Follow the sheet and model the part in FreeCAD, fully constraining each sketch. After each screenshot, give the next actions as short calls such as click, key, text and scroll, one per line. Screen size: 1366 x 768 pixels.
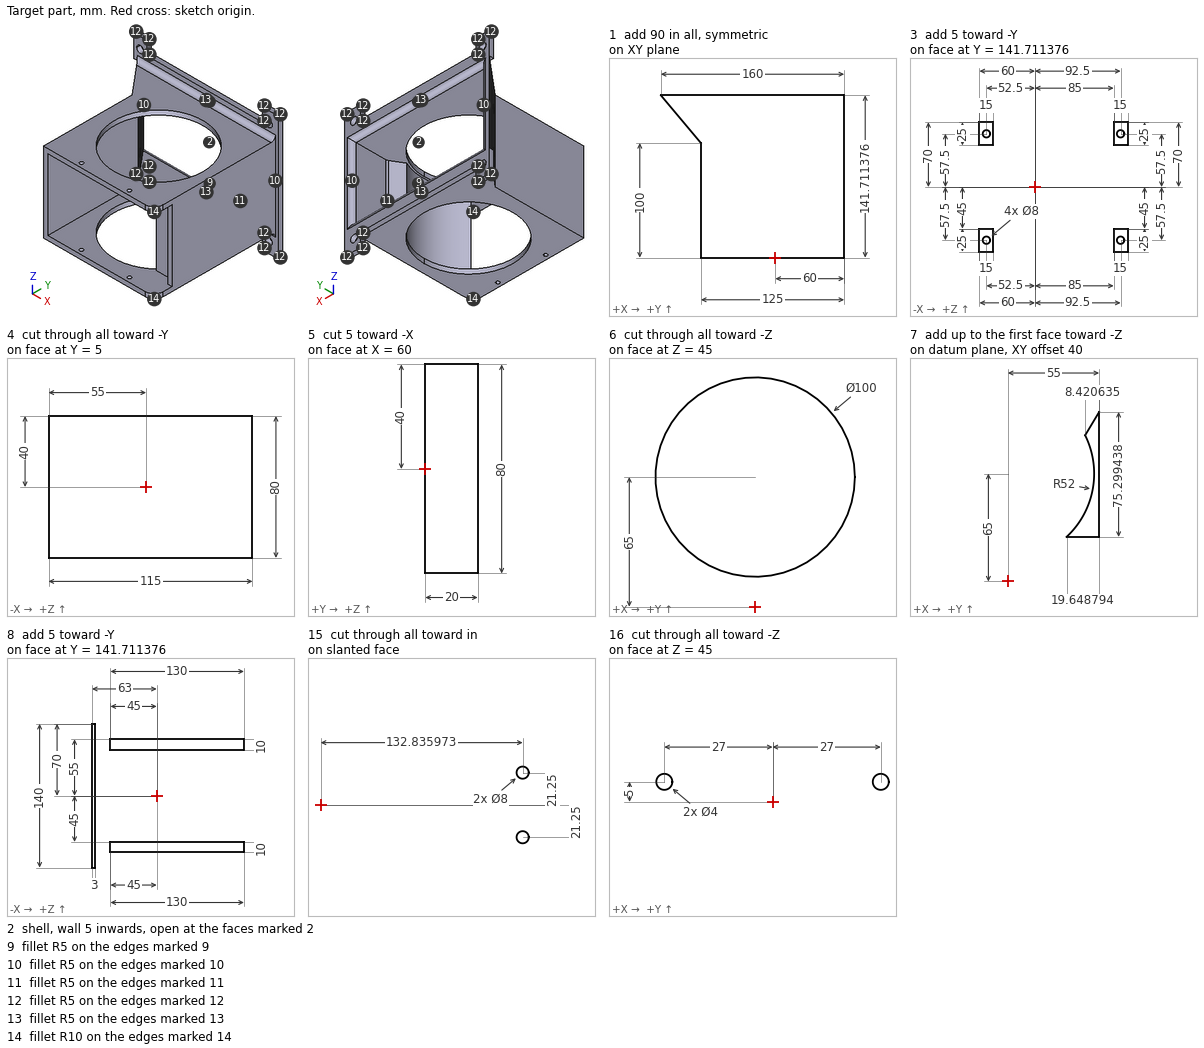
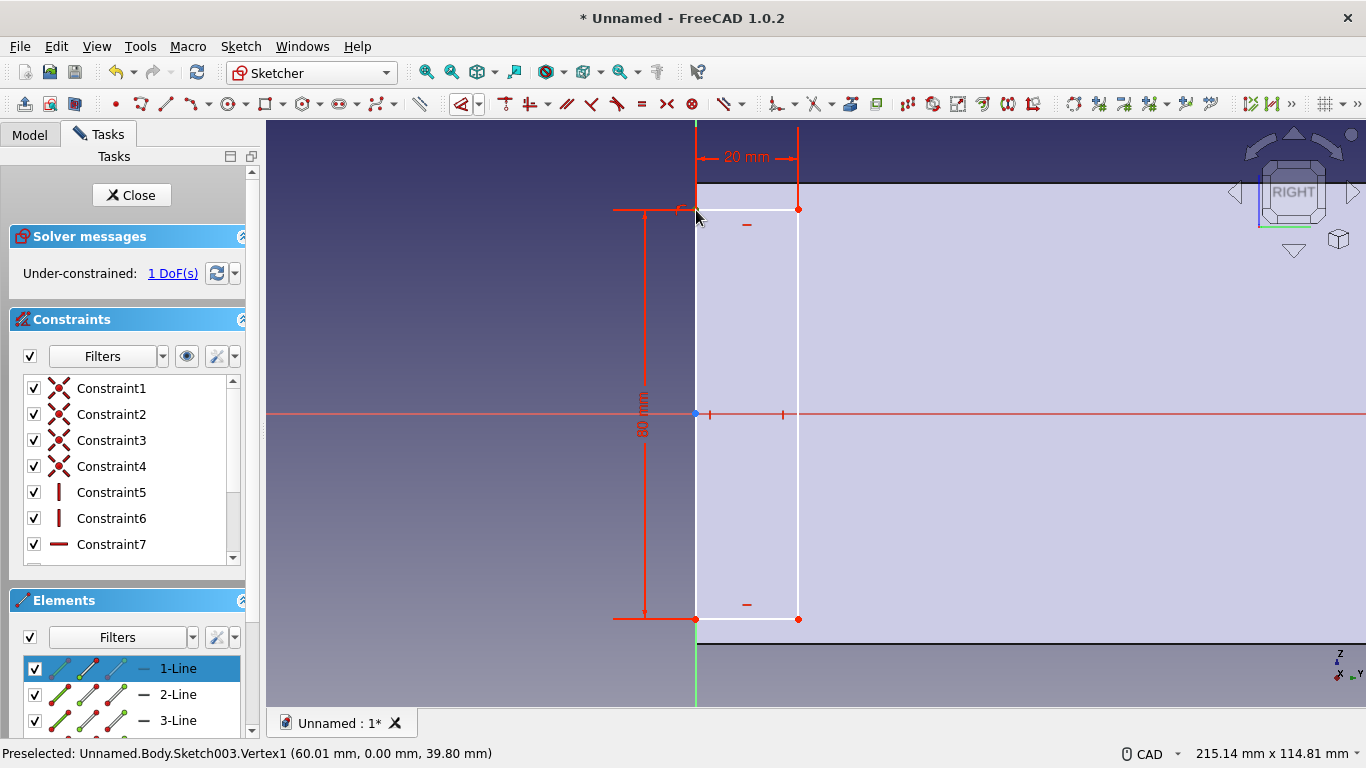
key(i)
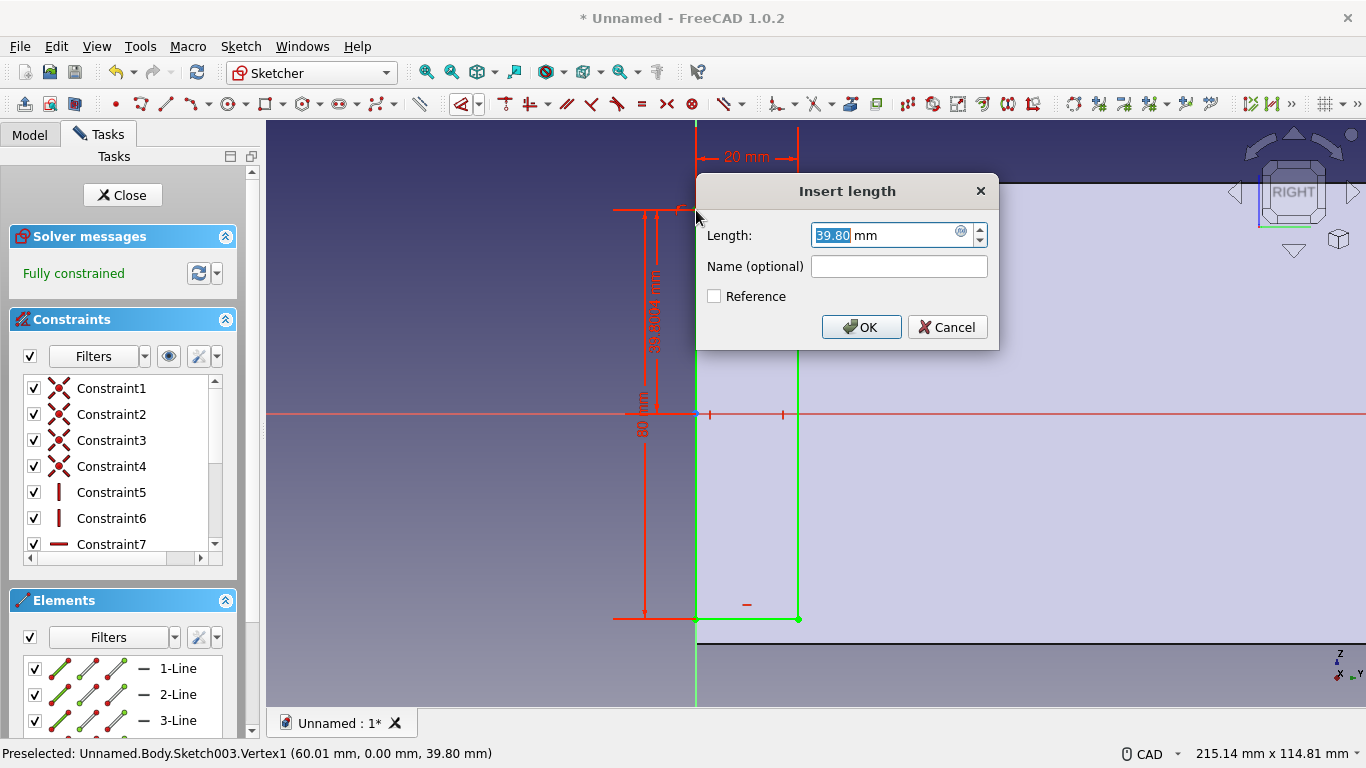
text(40)
key(Return)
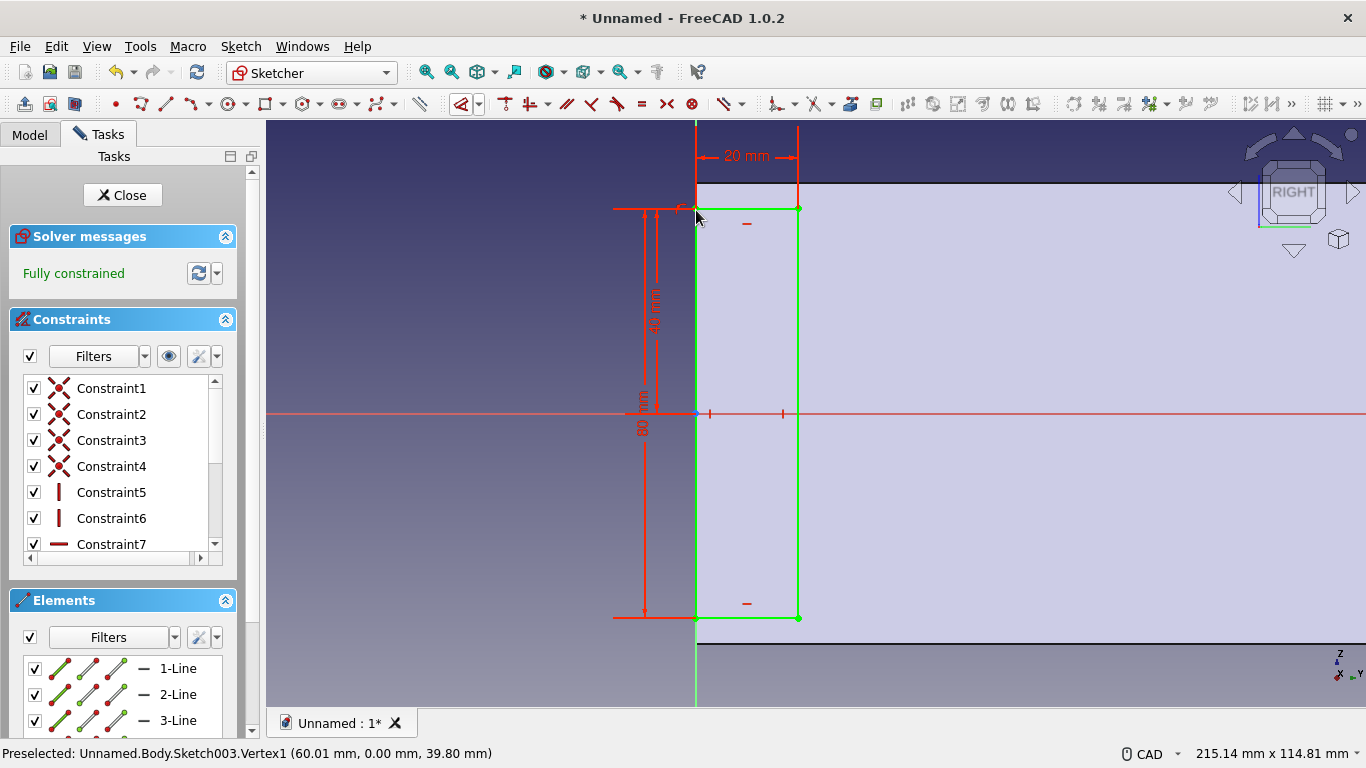
click(123, 195)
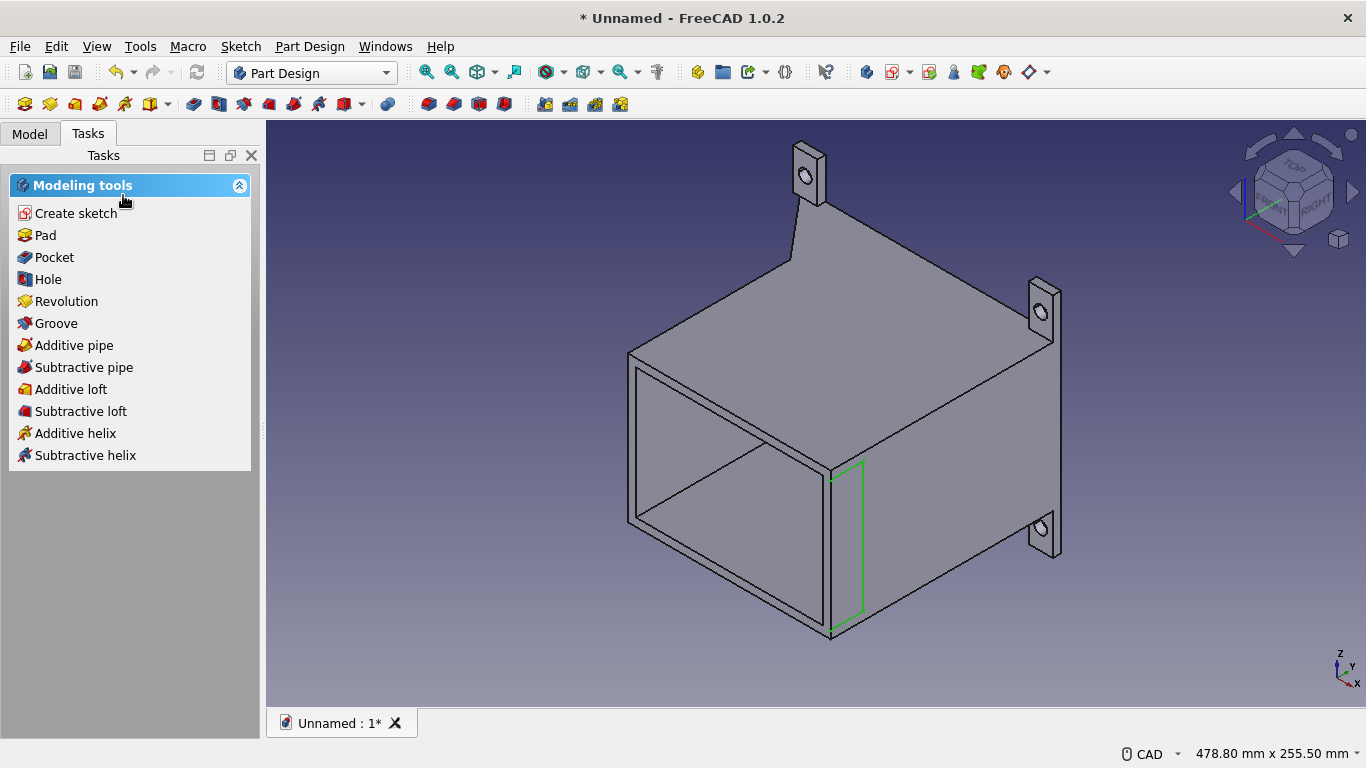
click(194, 104)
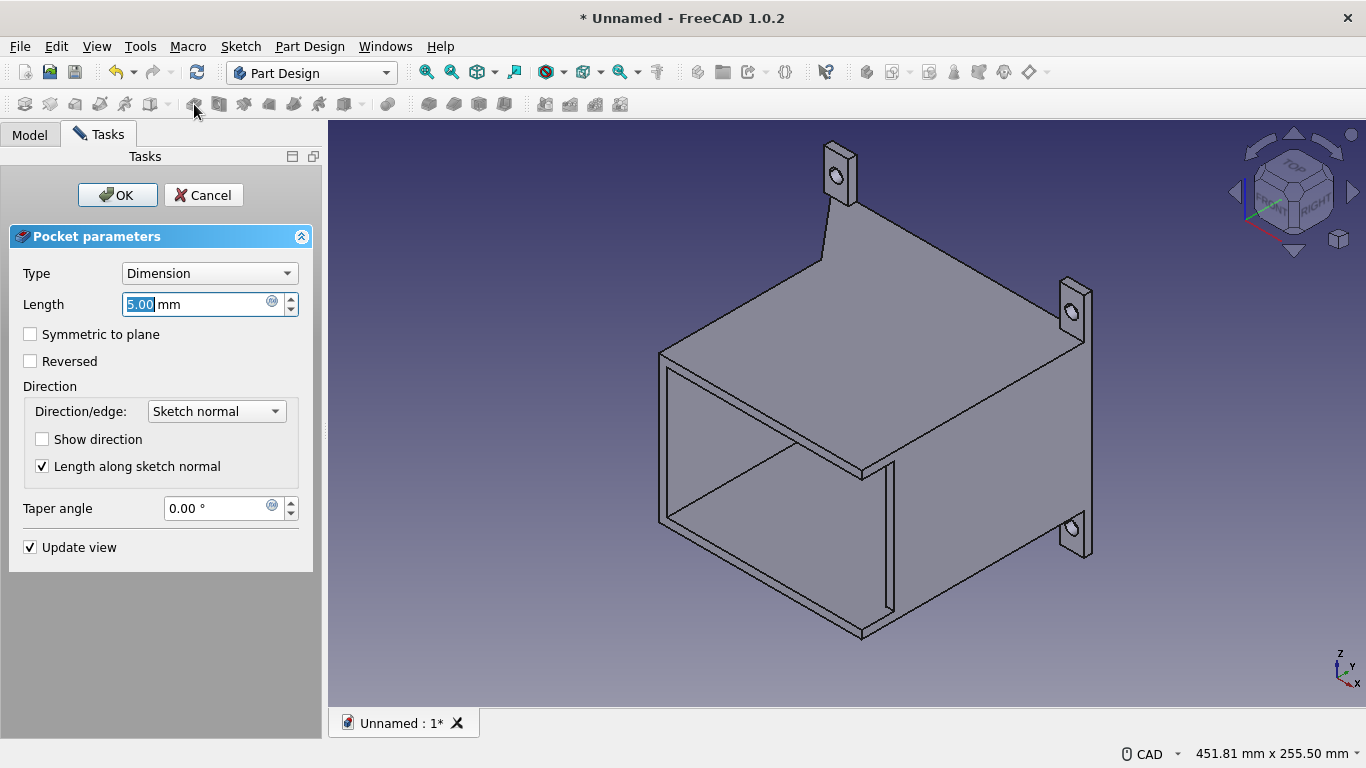
text(5)
key(Tab)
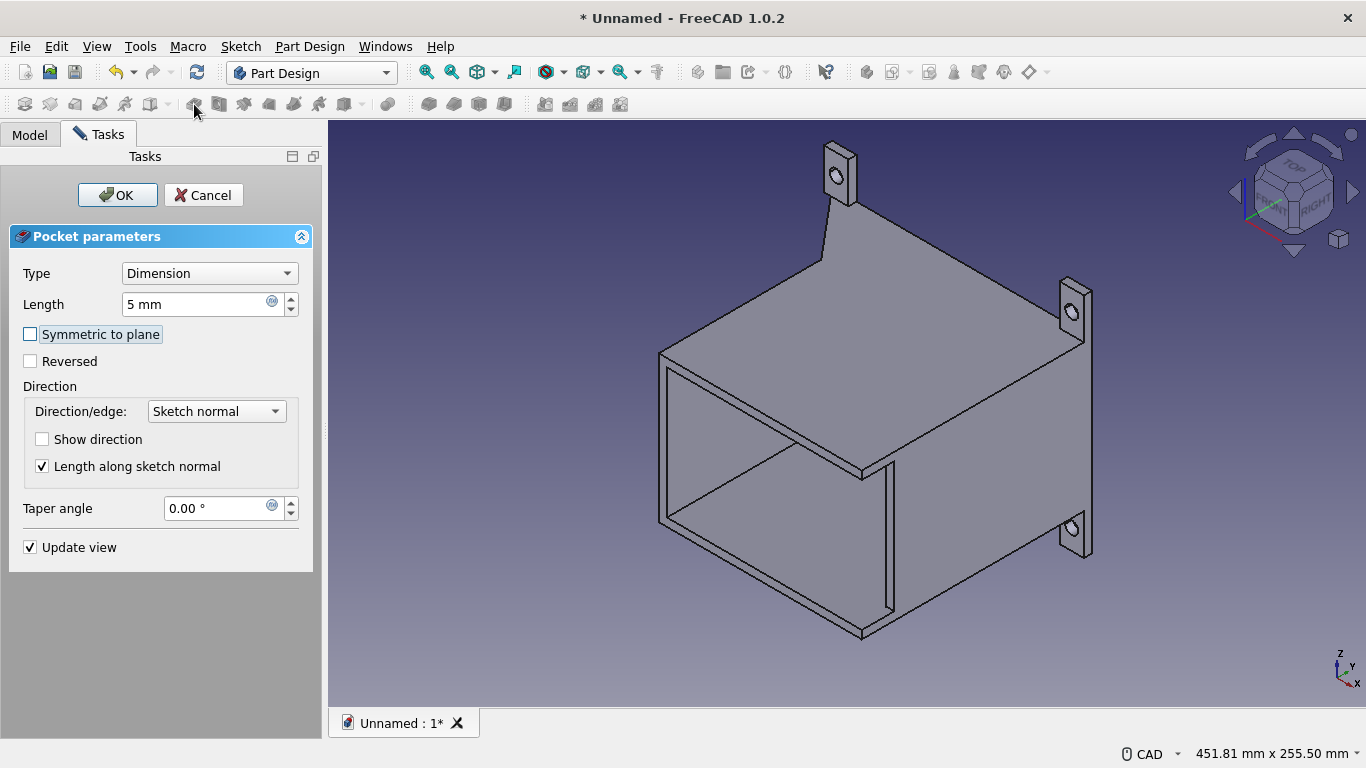
click(118, 195)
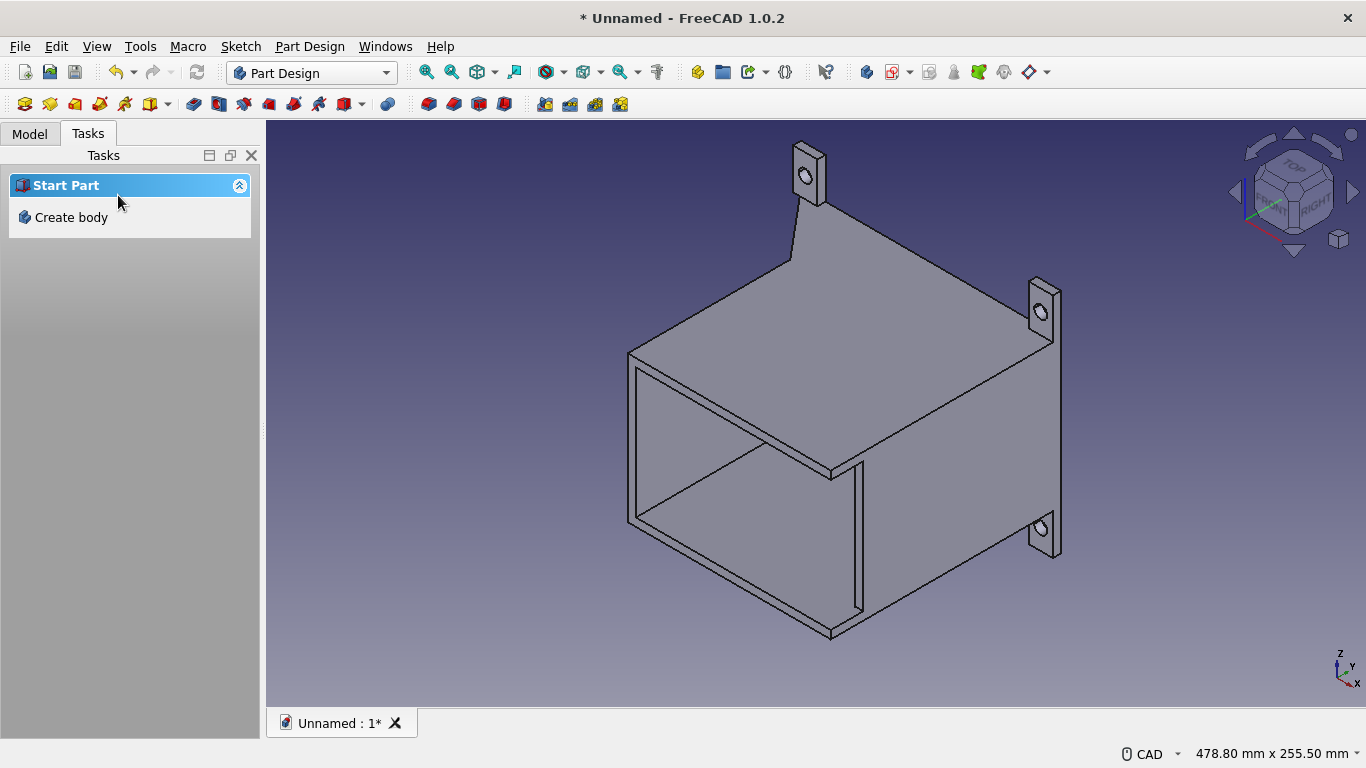
click(856, 351)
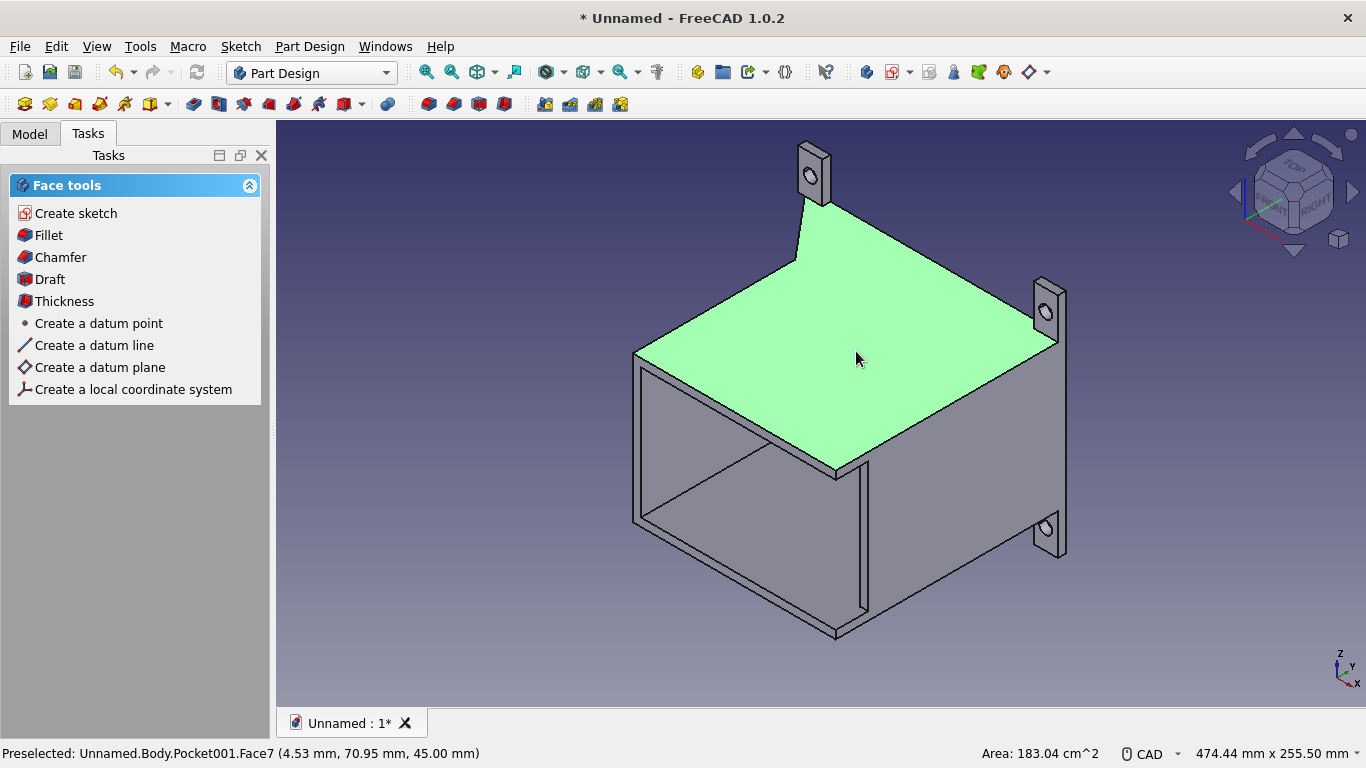
click(892, 72)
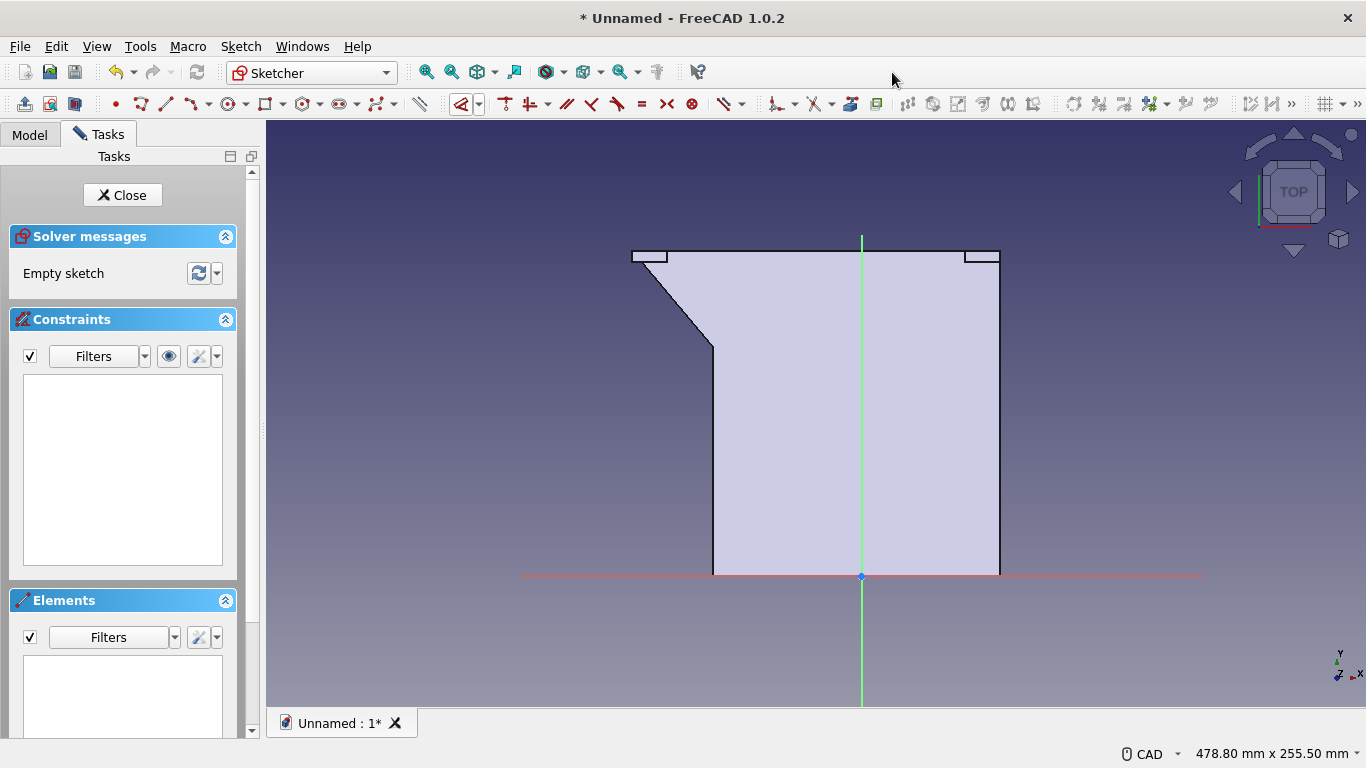
key(q)
key(s)